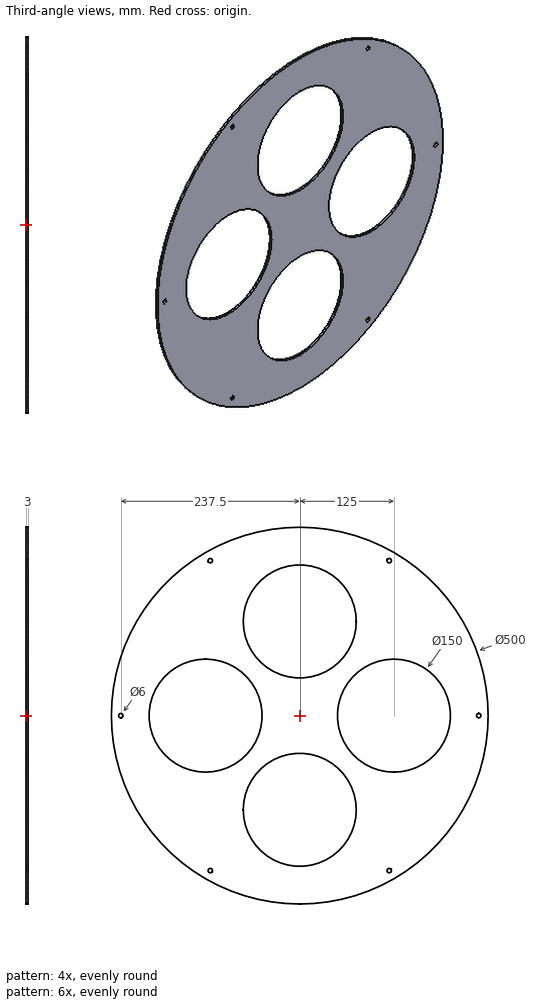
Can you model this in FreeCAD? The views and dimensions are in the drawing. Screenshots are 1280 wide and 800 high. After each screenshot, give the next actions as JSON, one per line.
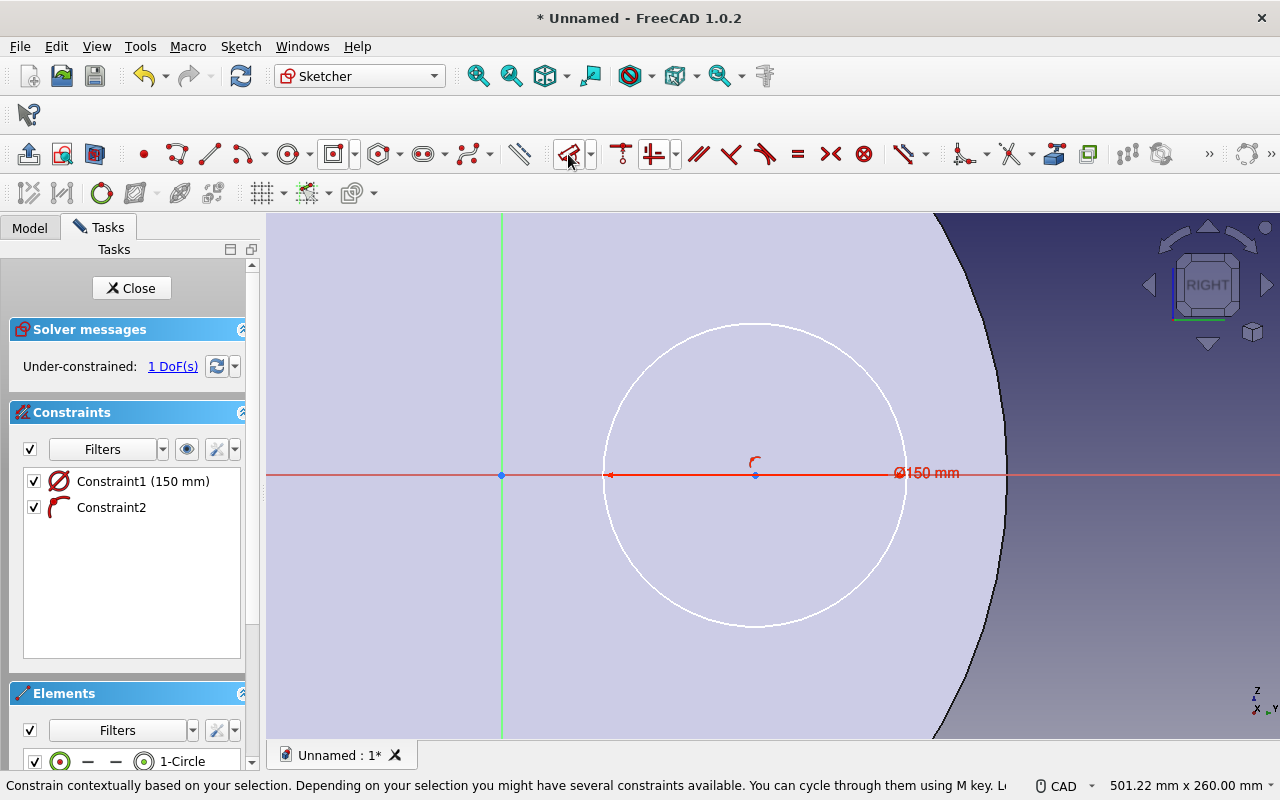
{"action": "left_click", "coordinate": [755, 475]}
{"action": "left_click", "coordinate": [628, 509]}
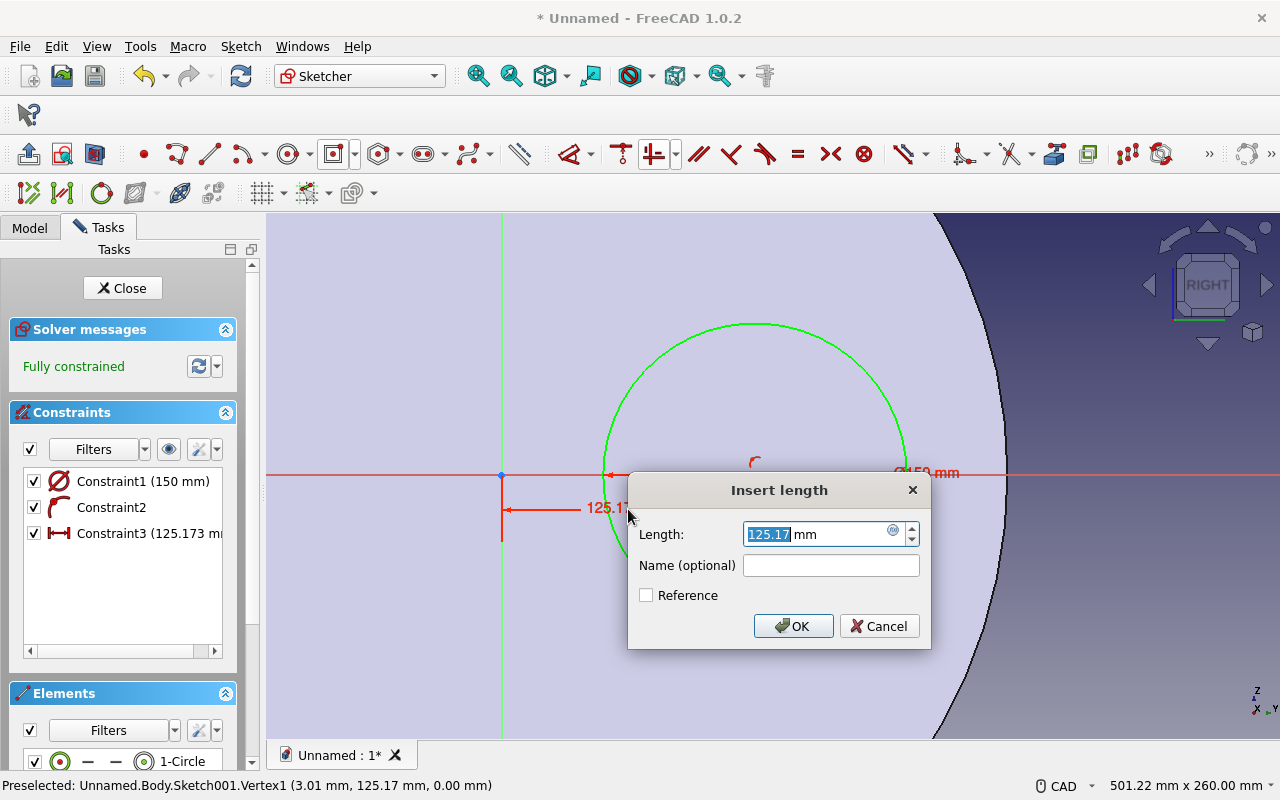
{"action": "type", "text": "125"}
{"action": "key", "text": "Return"}
{"action": "key", "text": "Escape"}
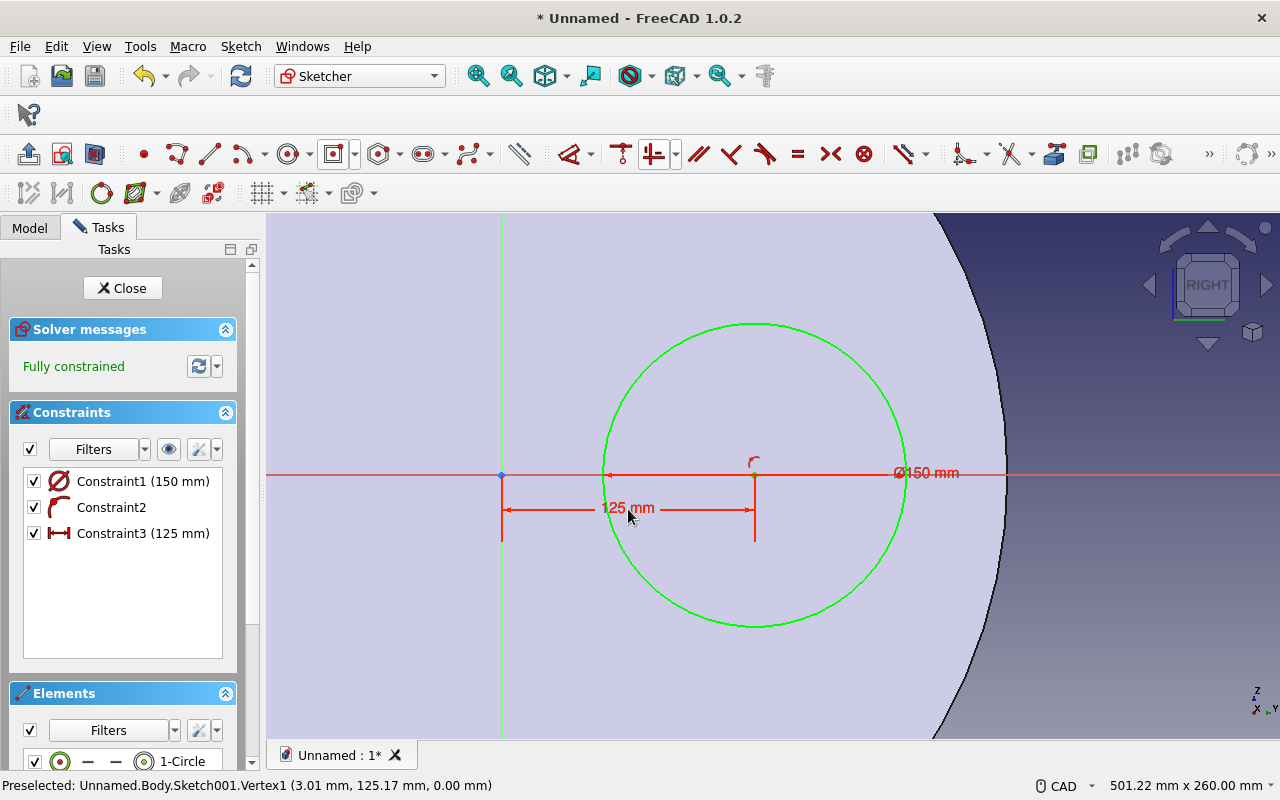
{"action": "left_click", "coordinate": [123, 288]}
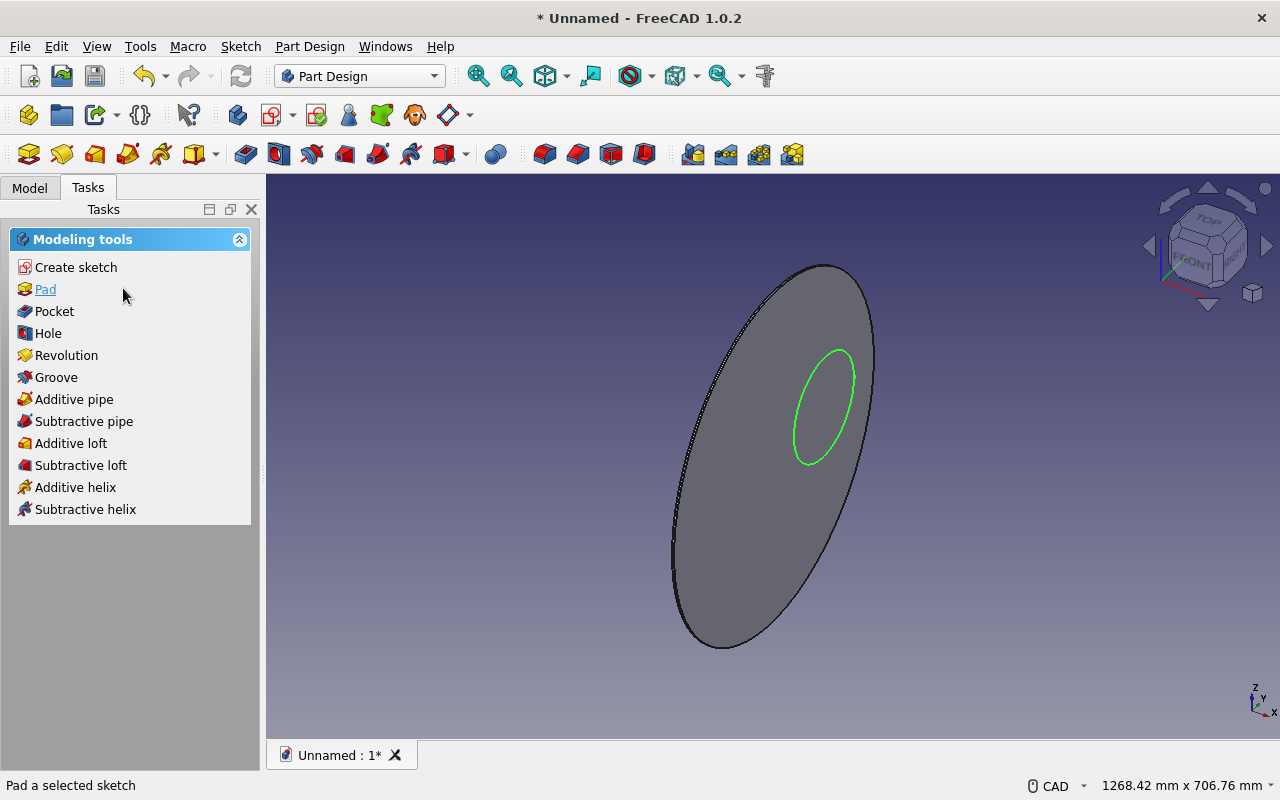
{"action": "left_click", "coordinate": [246, 154]}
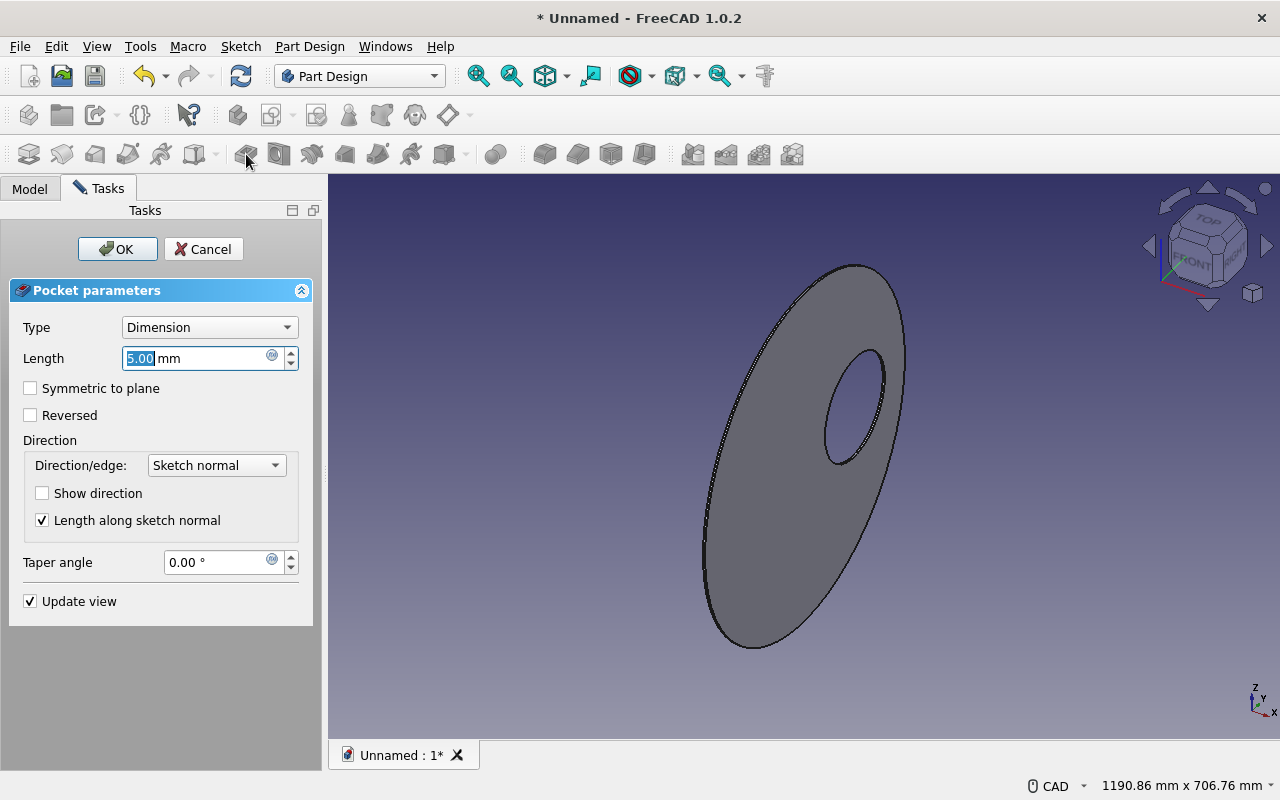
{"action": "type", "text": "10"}
{"action": "key", "text": "Tab"}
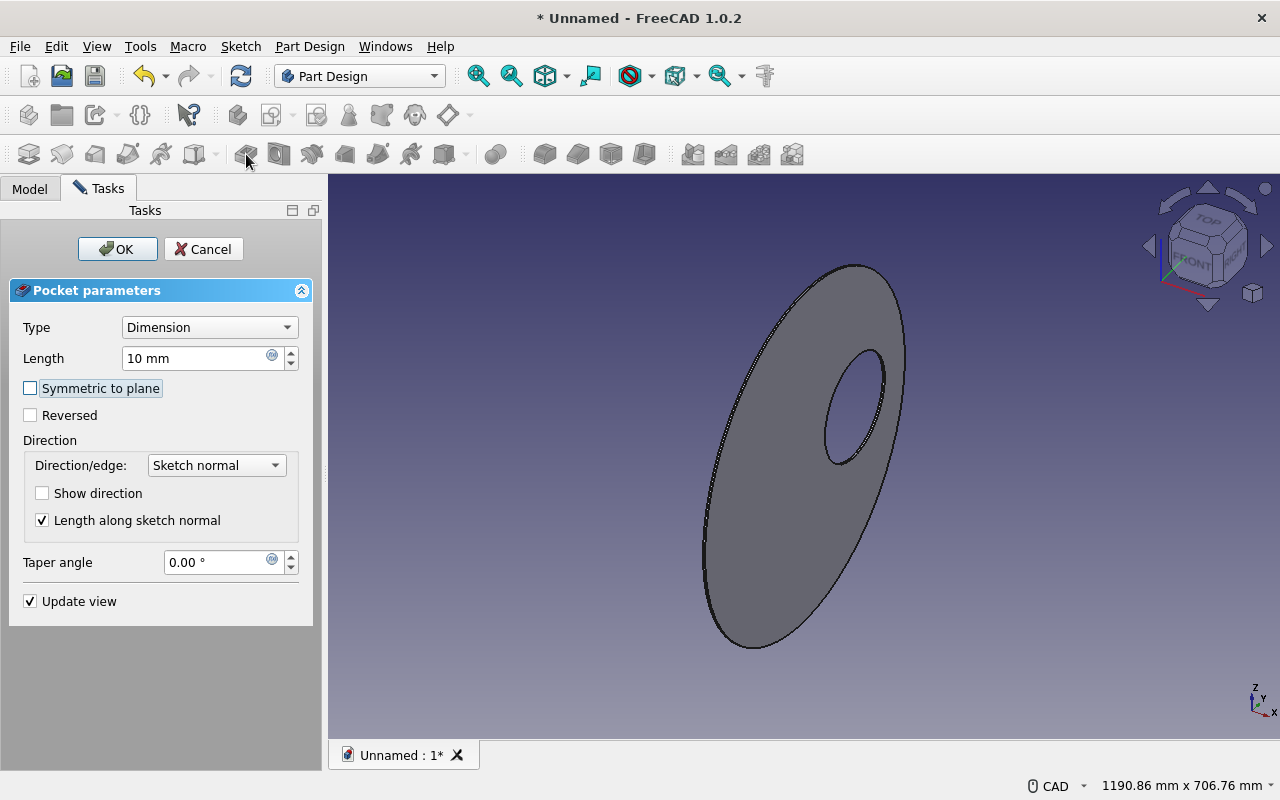
{"action": "left_click", "coordinate": [118, 249]}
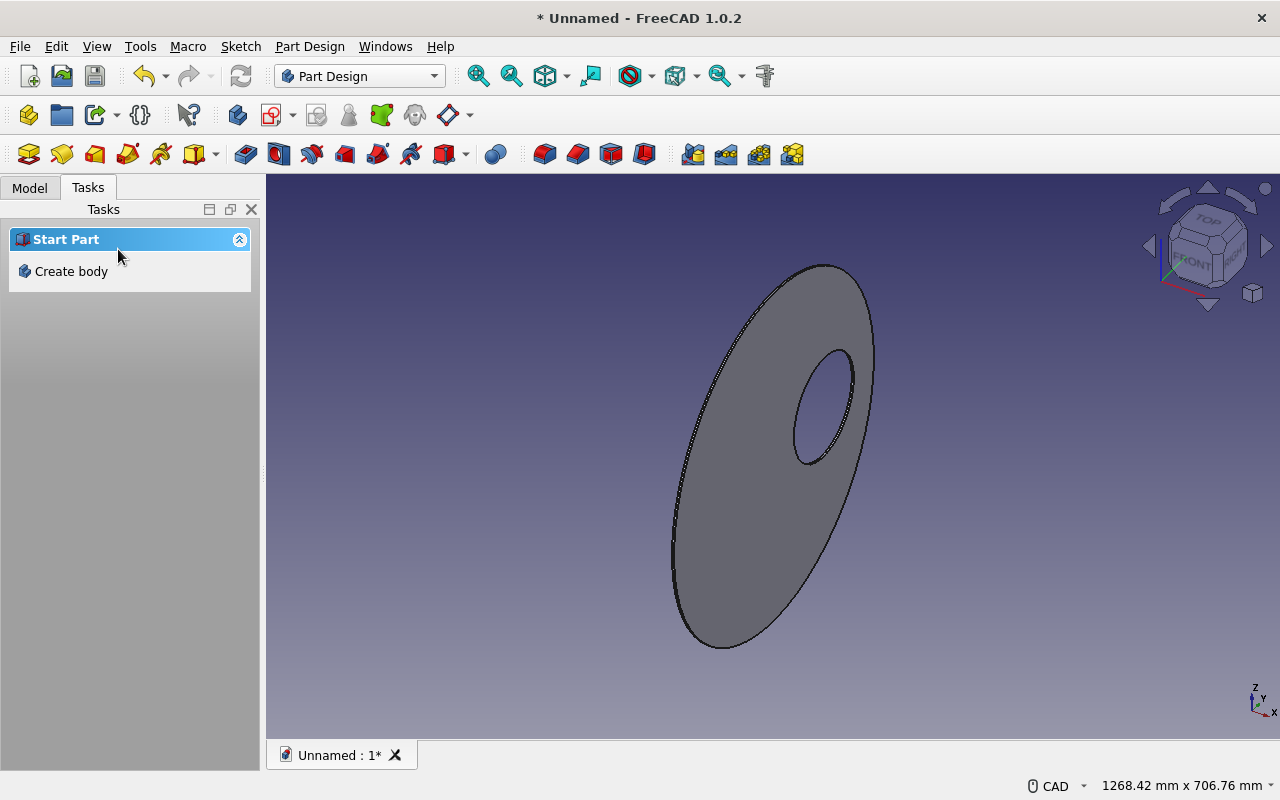
{"action": "left_click", "coordinate": [30, 188]}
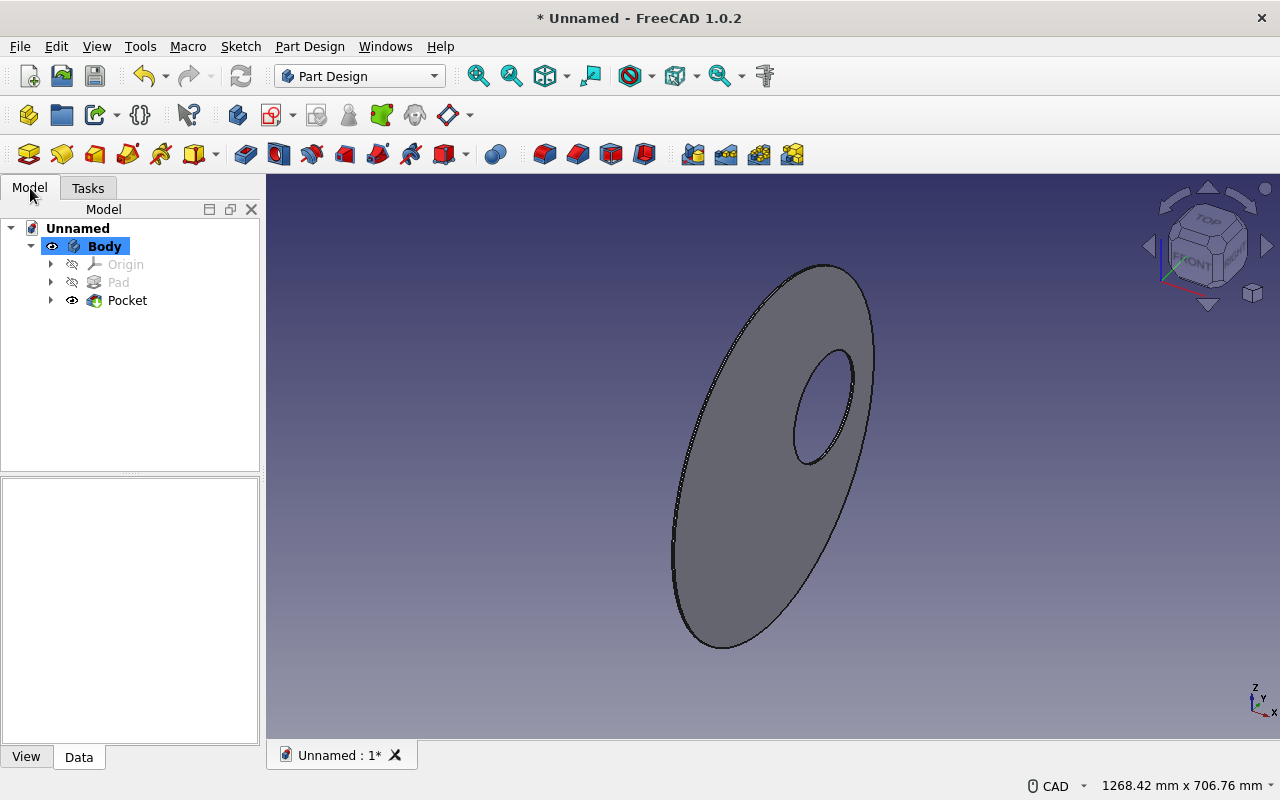
{"action": "left_click", "coordinate": [117, 300]}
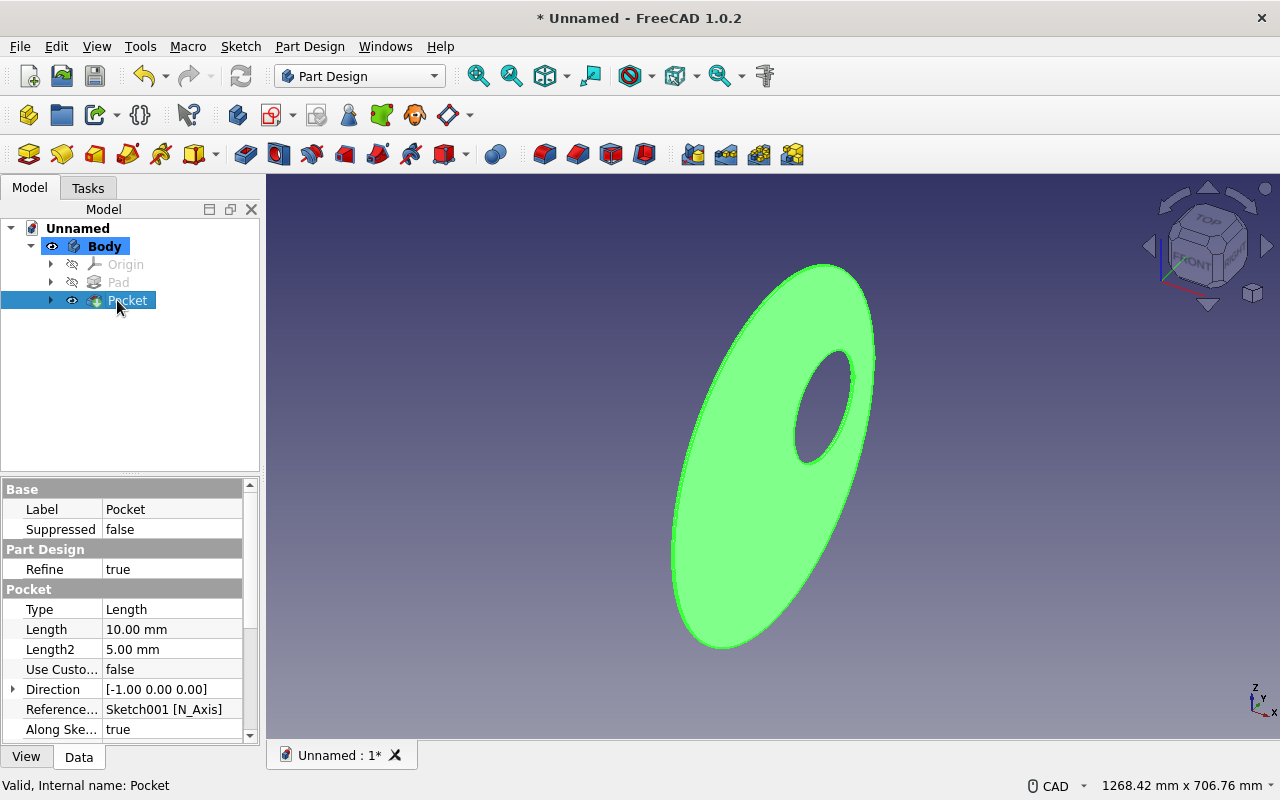
{"action": "left_click", "coordinate": [759, 154]}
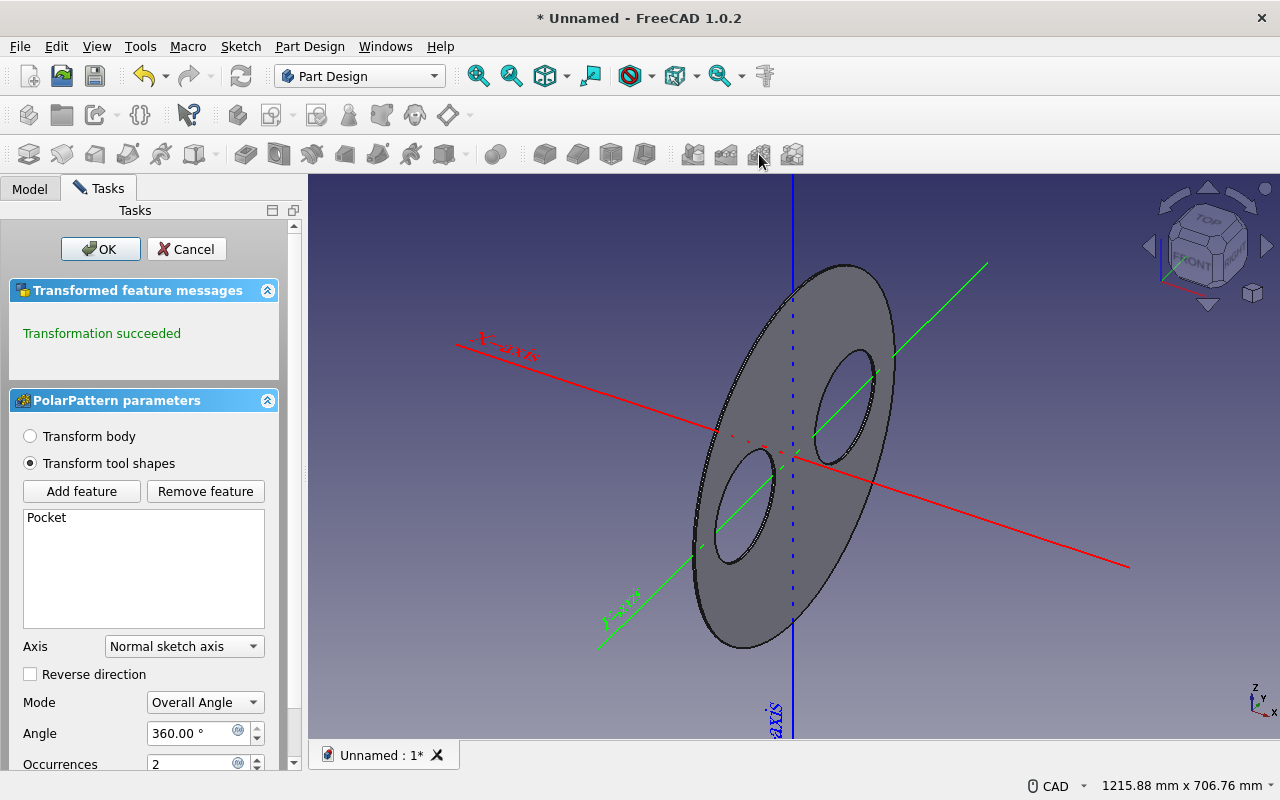
{"action": "left_click", "coordinate": [185, 646]}